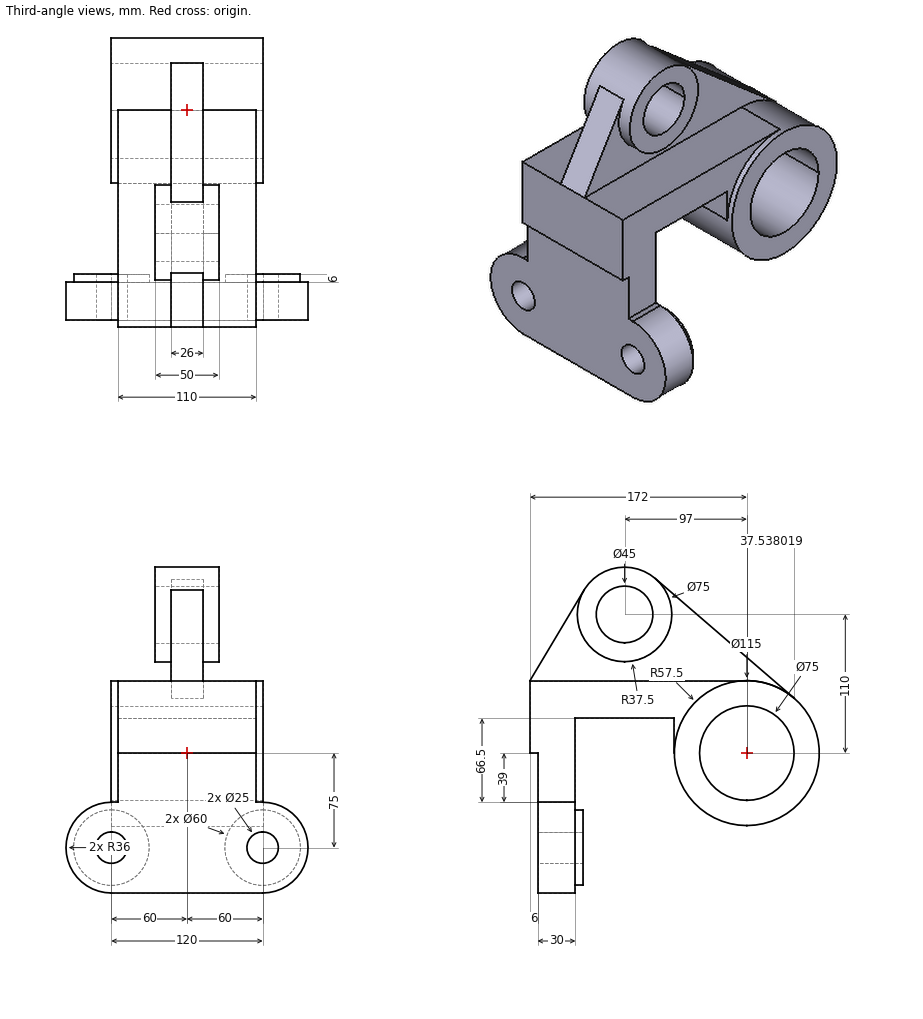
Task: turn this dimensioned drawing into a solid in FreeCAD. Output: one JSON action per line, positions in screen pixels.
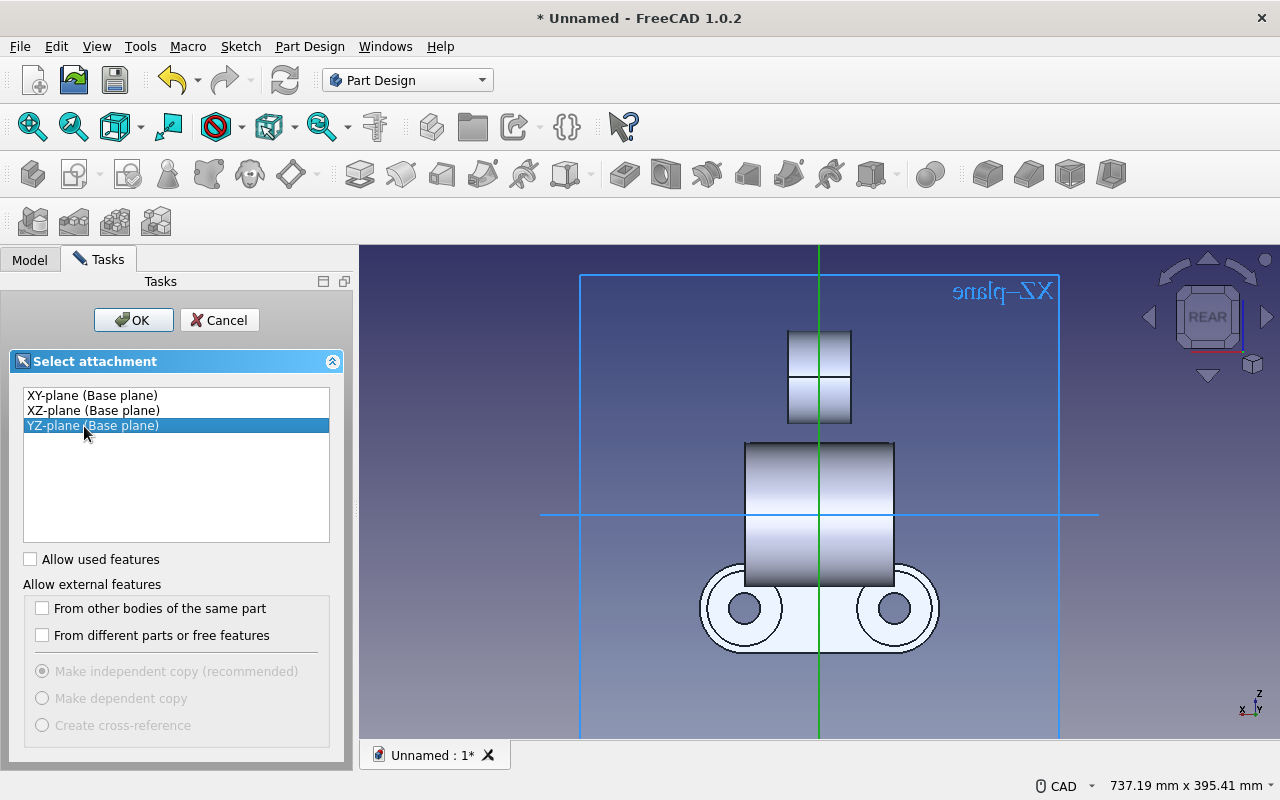
{"action": "left_click", "coordinate": [134, 320]}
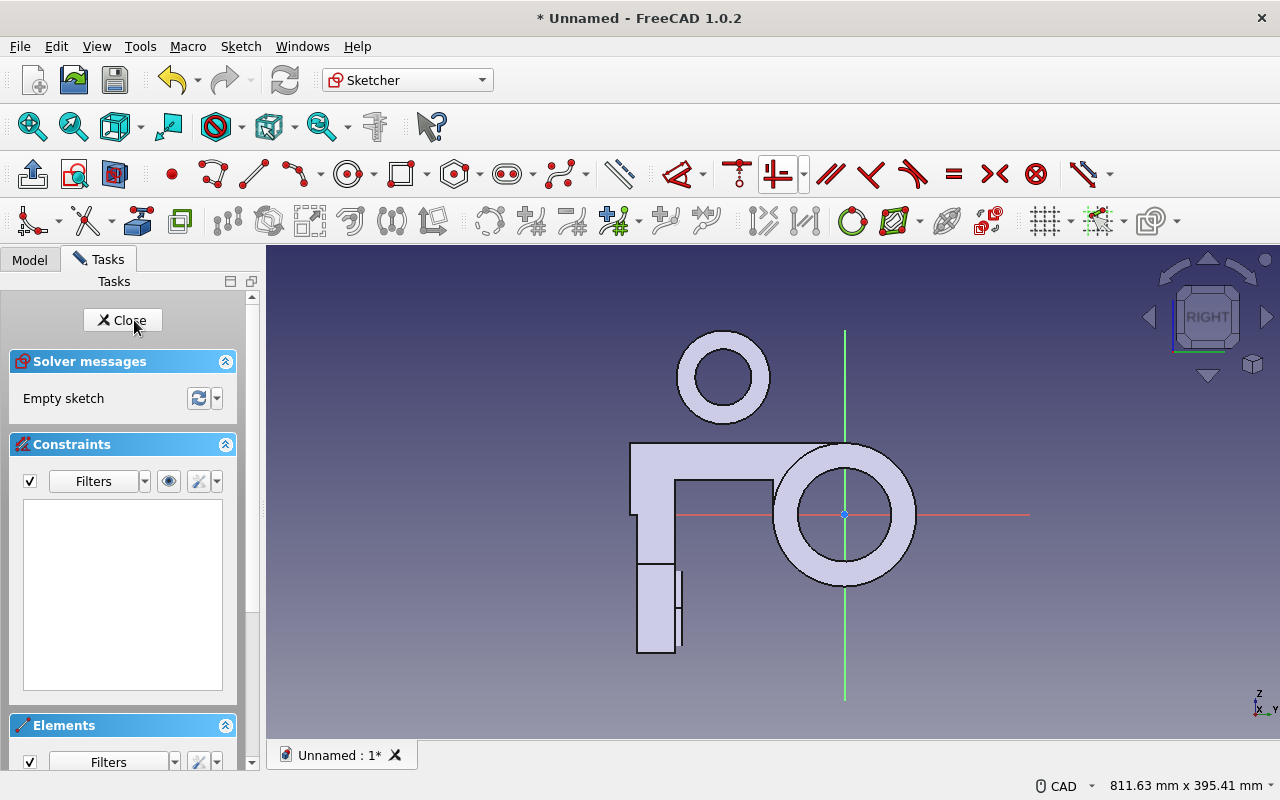
{"action": "left_click", "coordinate": [115, 174]}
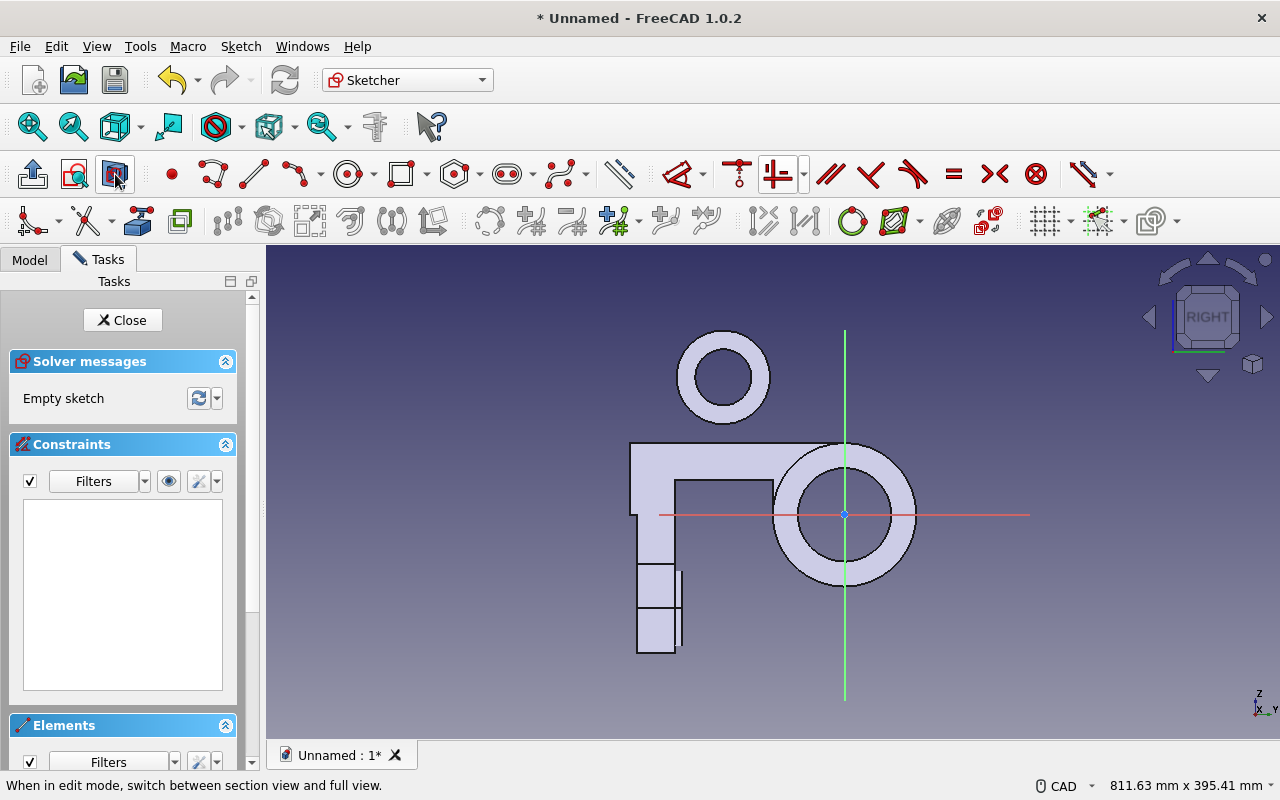
{"action": "scroll", "coordinate": [829, 351], "scroll_direction": "up", "scroll_amount": 3}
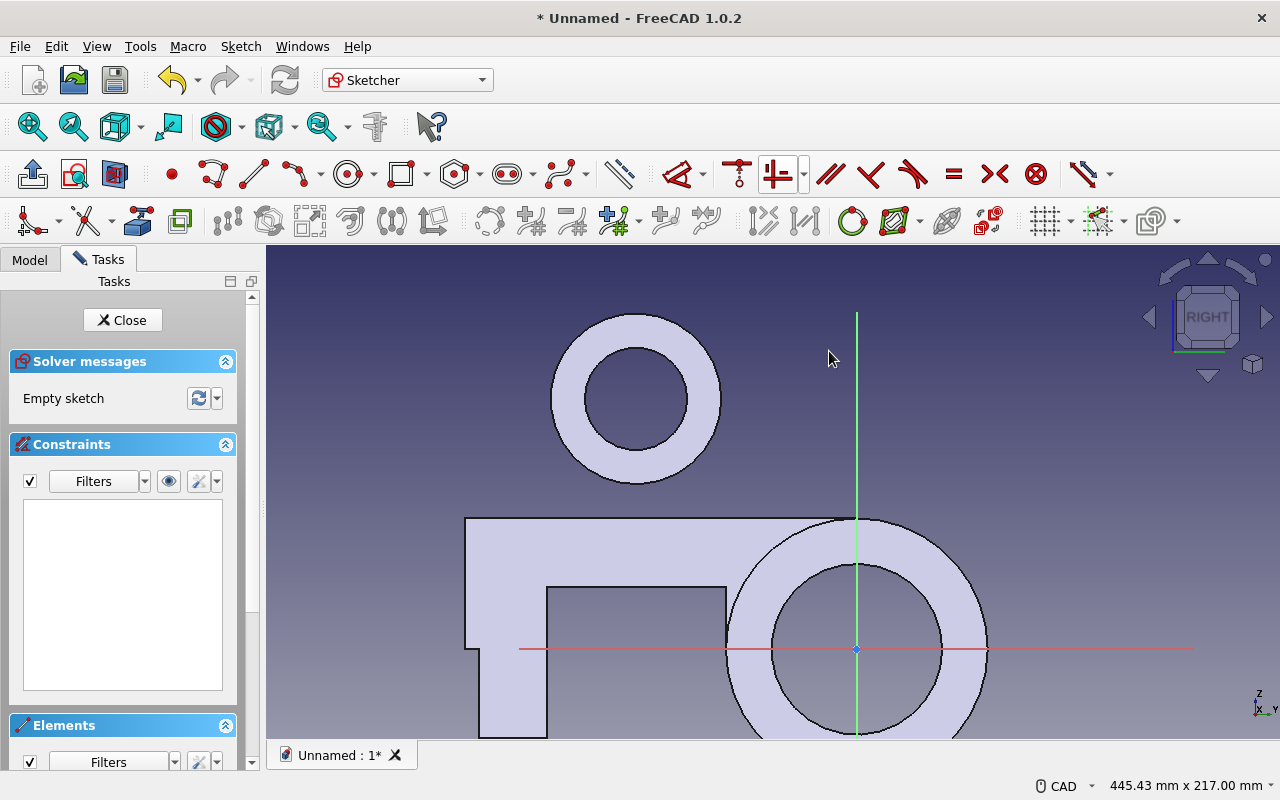
{"action": "key", "text": "g l"}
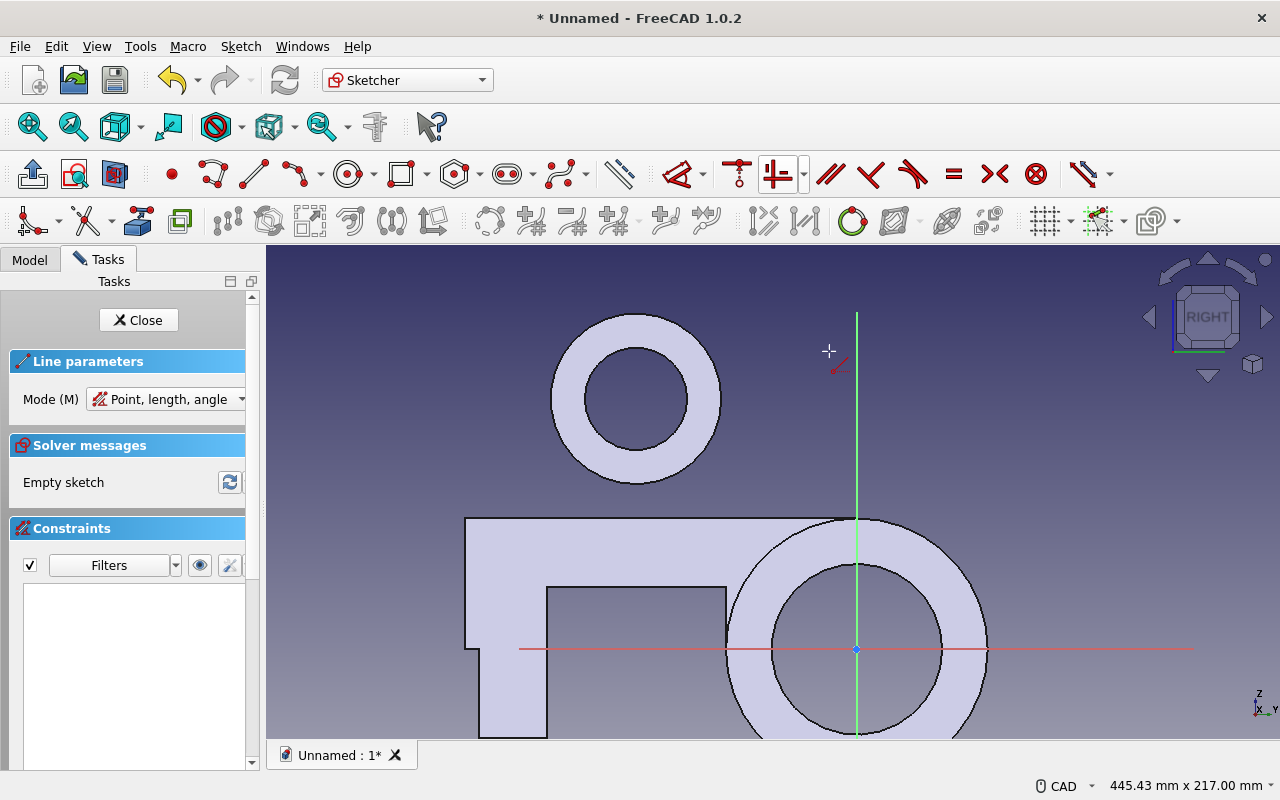
{"action": "left_click", "coordinate": [942, 550]}
{"action": "left_click", "coordinate": [692, 334]}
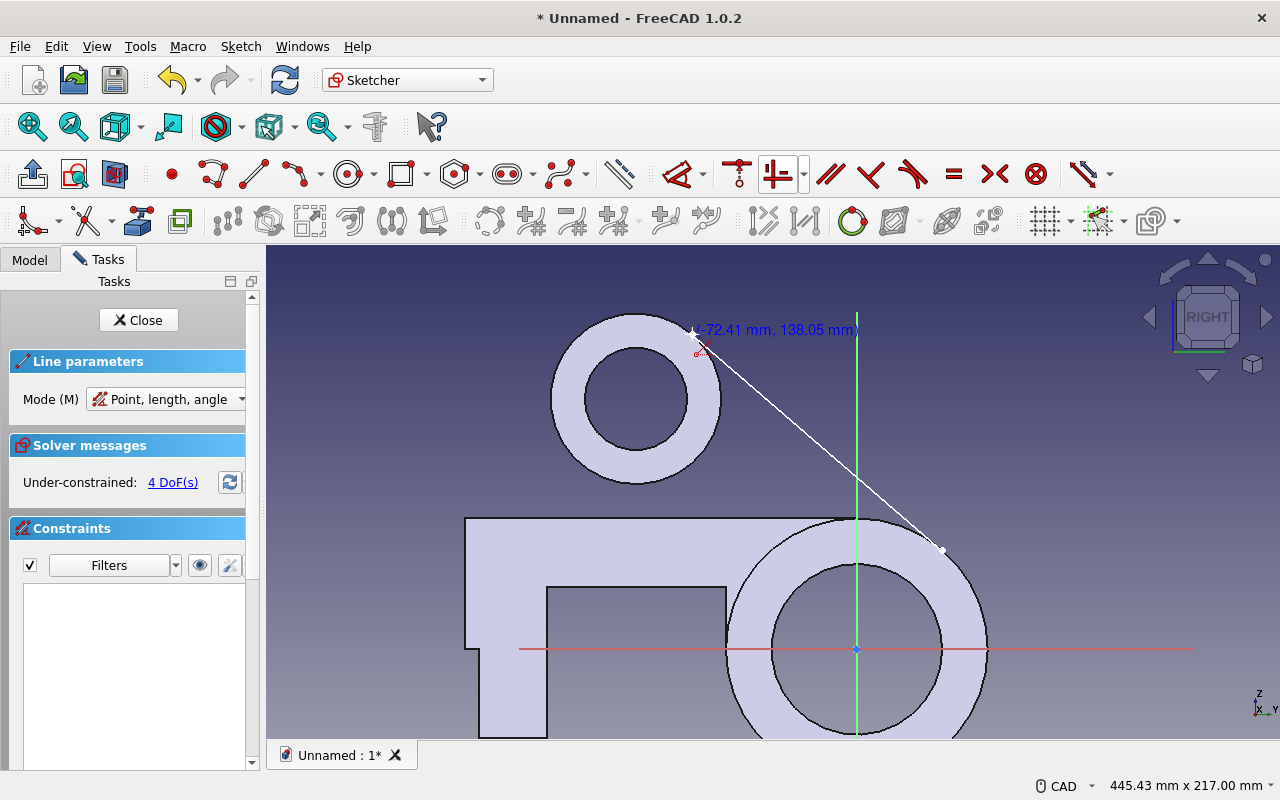
{"action": "left_click", "coordinate": [213, 174]}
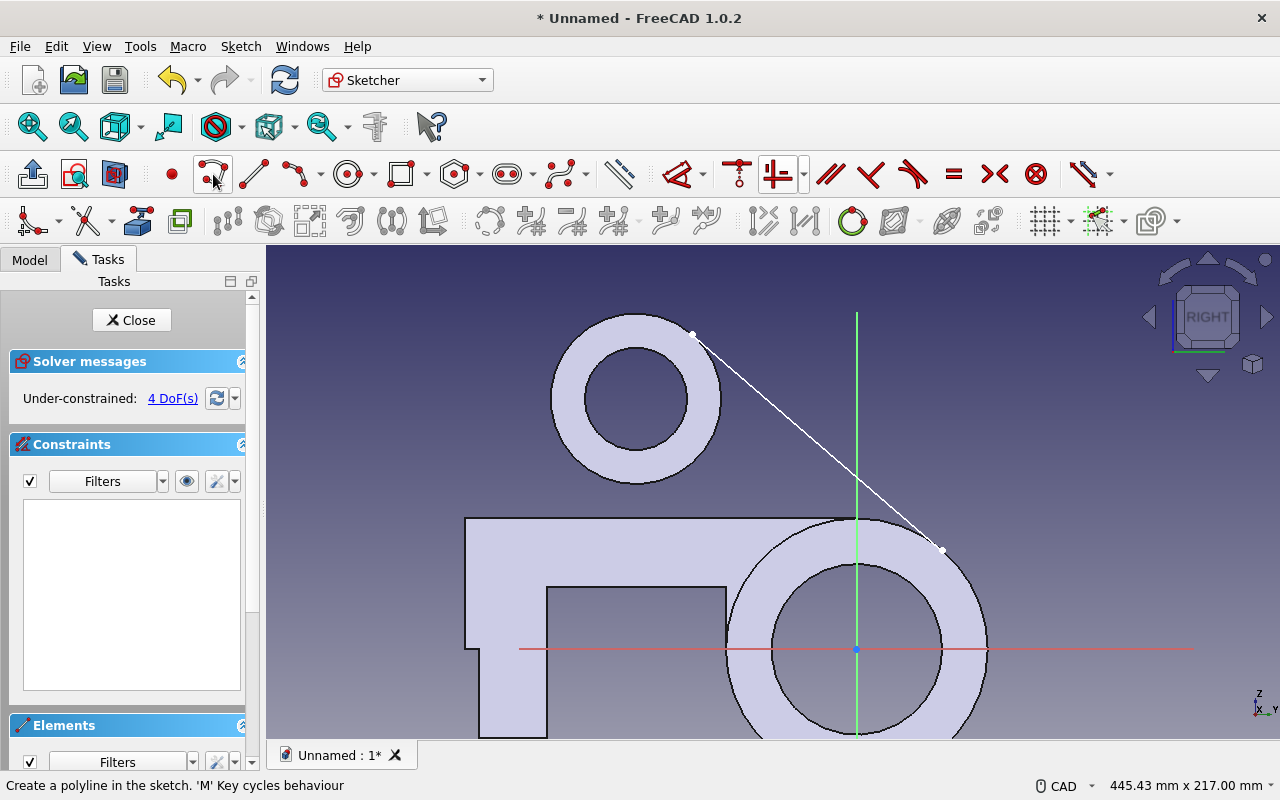
{"action": "left_click", "coordinate": [563, 355]}
{"action": "left_click", "coordinate": [465, 518]}
{"action": "left_click", "coordinate": [857, 518]}
{"action": "right_click", "coordinate": [857, 518]}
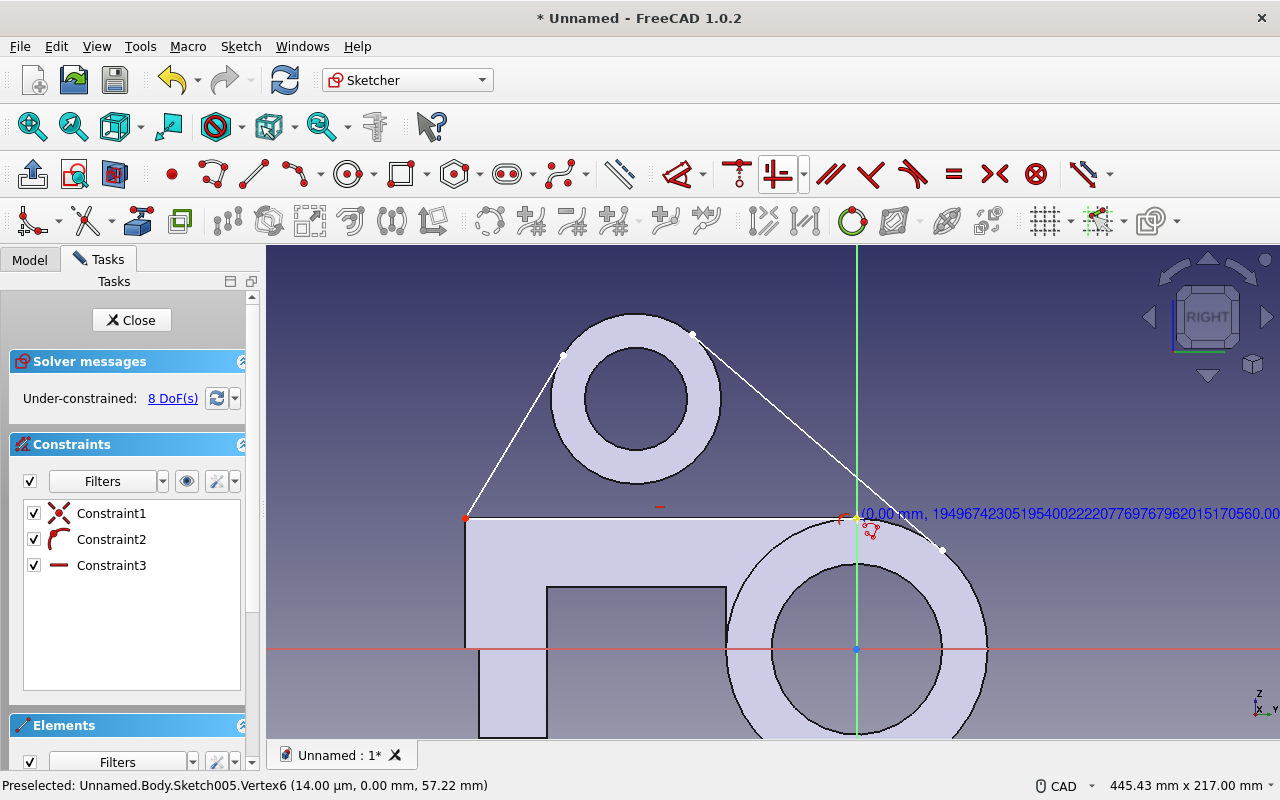
{"action": "left_click", "coordinate": [294, 174]}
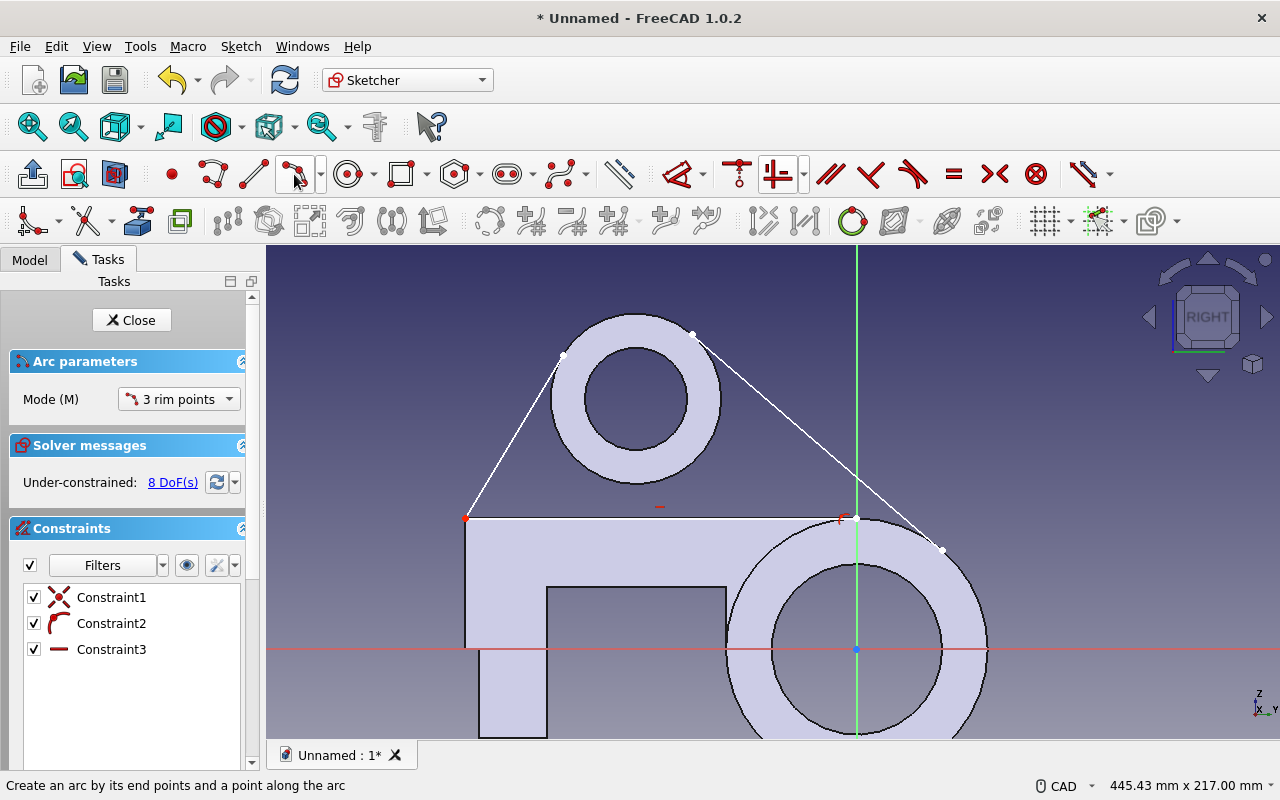
{"action": "left_click", "coordinate": [692, 335]}
{"action": "left_click", "coordinate": [563, 356]}
{"action": "left_click", "coordinate": [650, 483]}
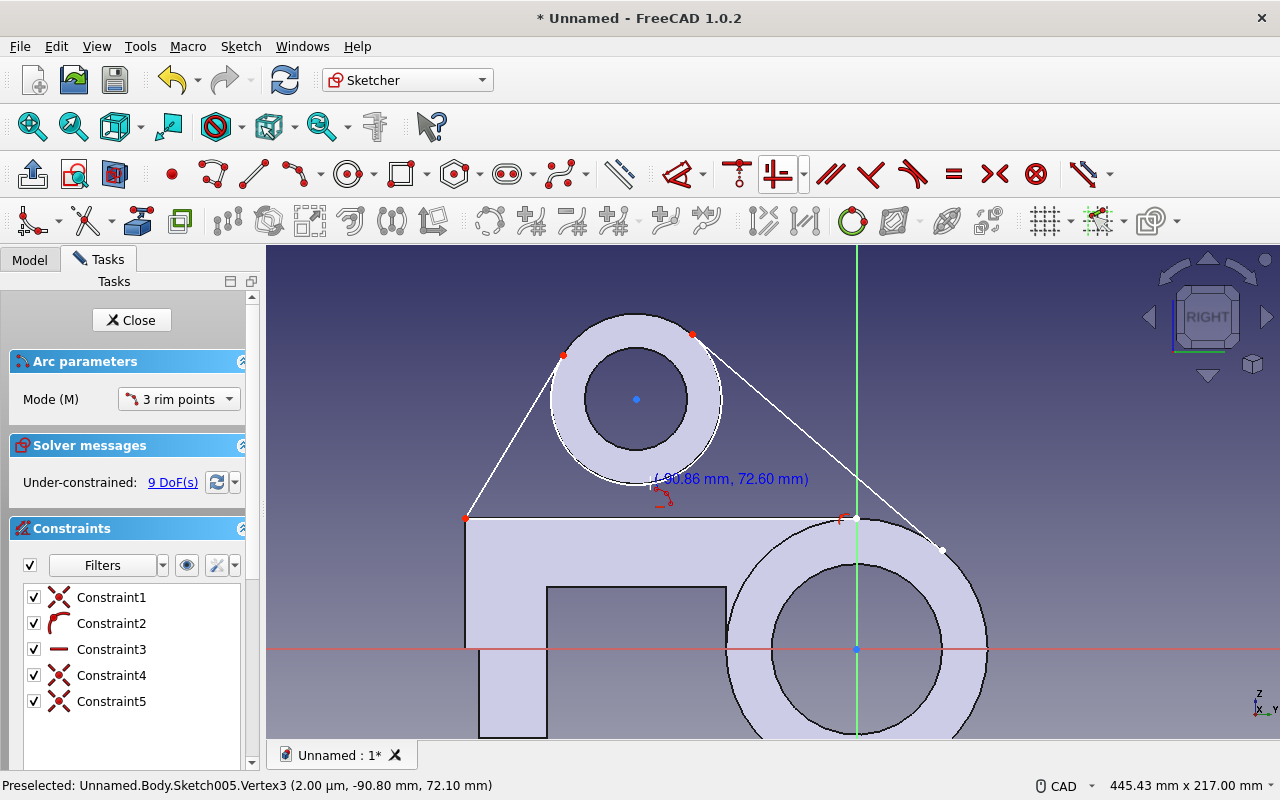
{"action": "left_click", "coordinate": [857, 519]}
{"action": "left_click", "coordinate": [942, 551]}